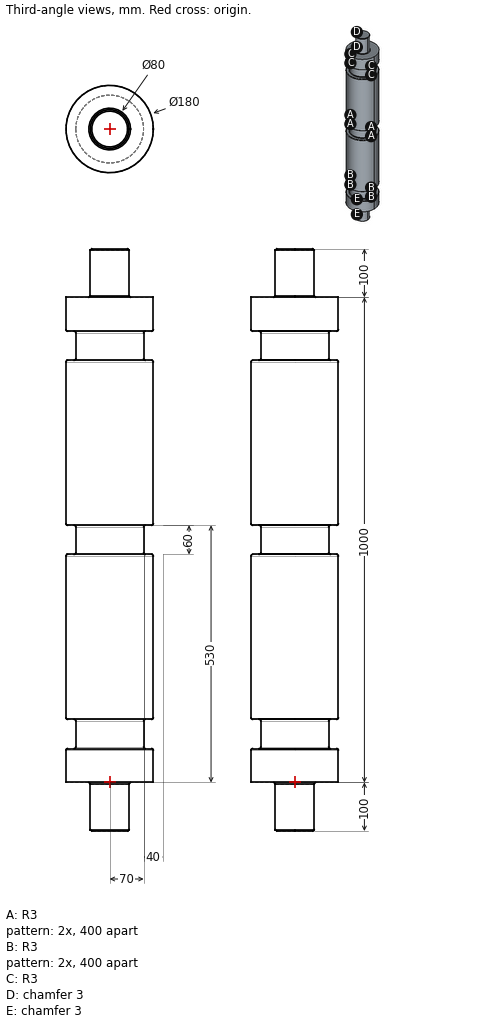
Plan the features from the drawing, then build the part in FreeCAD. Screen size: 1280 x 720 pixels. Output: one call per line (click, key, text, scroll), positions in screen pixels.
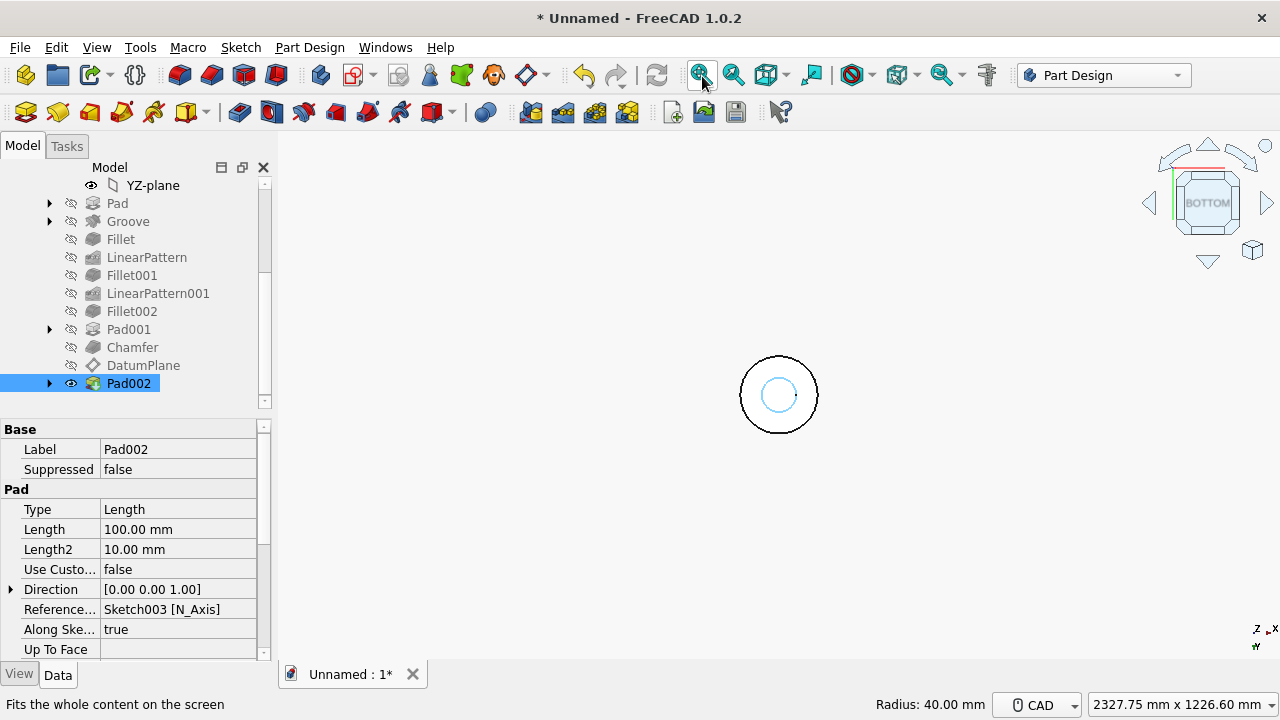
click(702, 76)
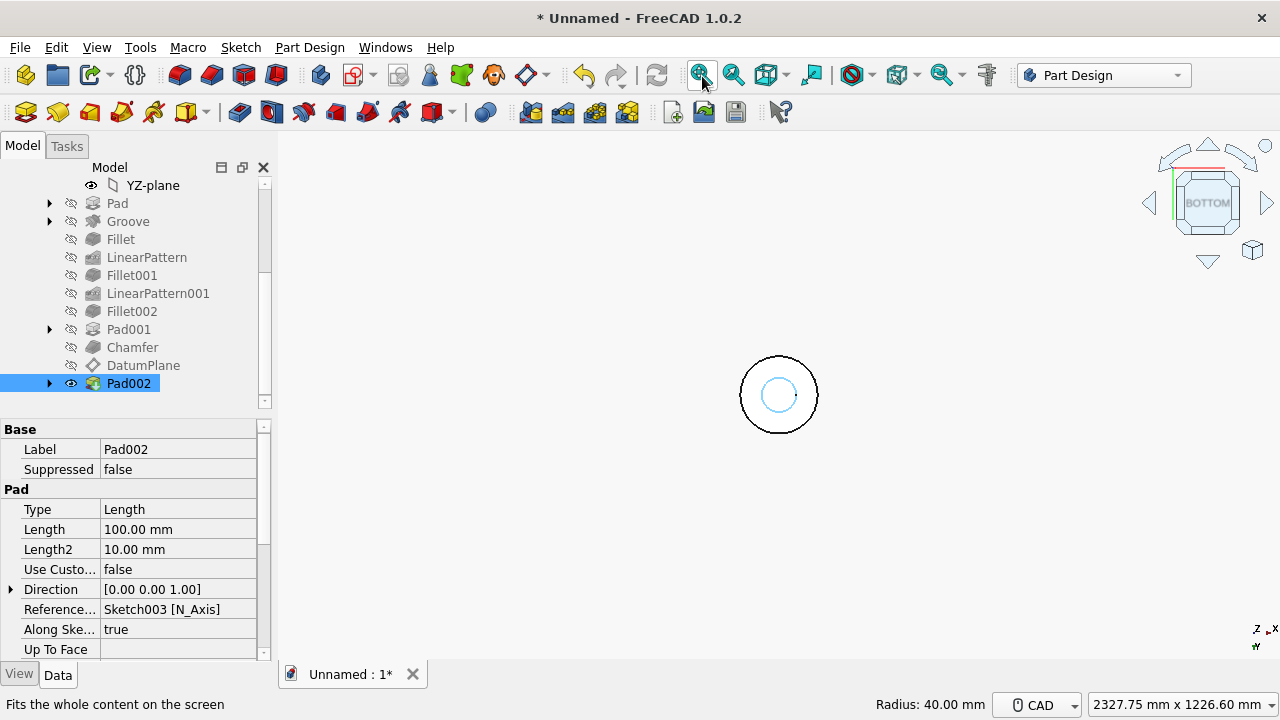
key(4)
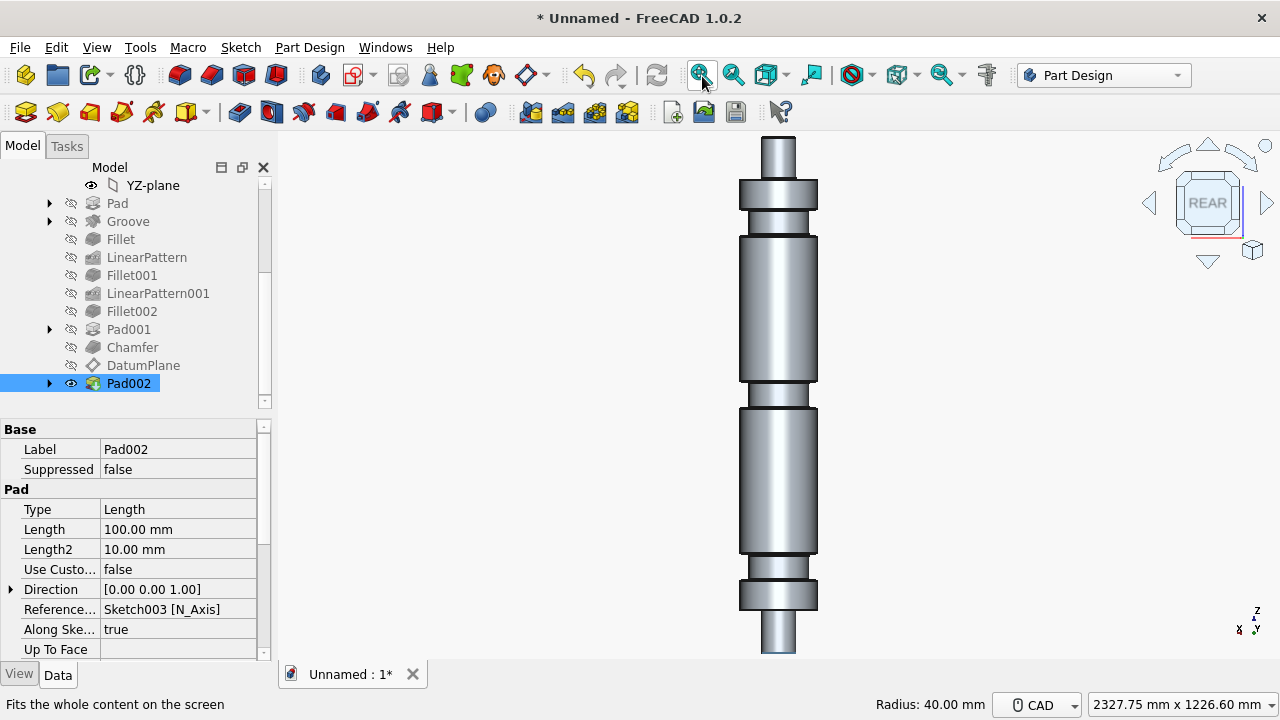
key(6)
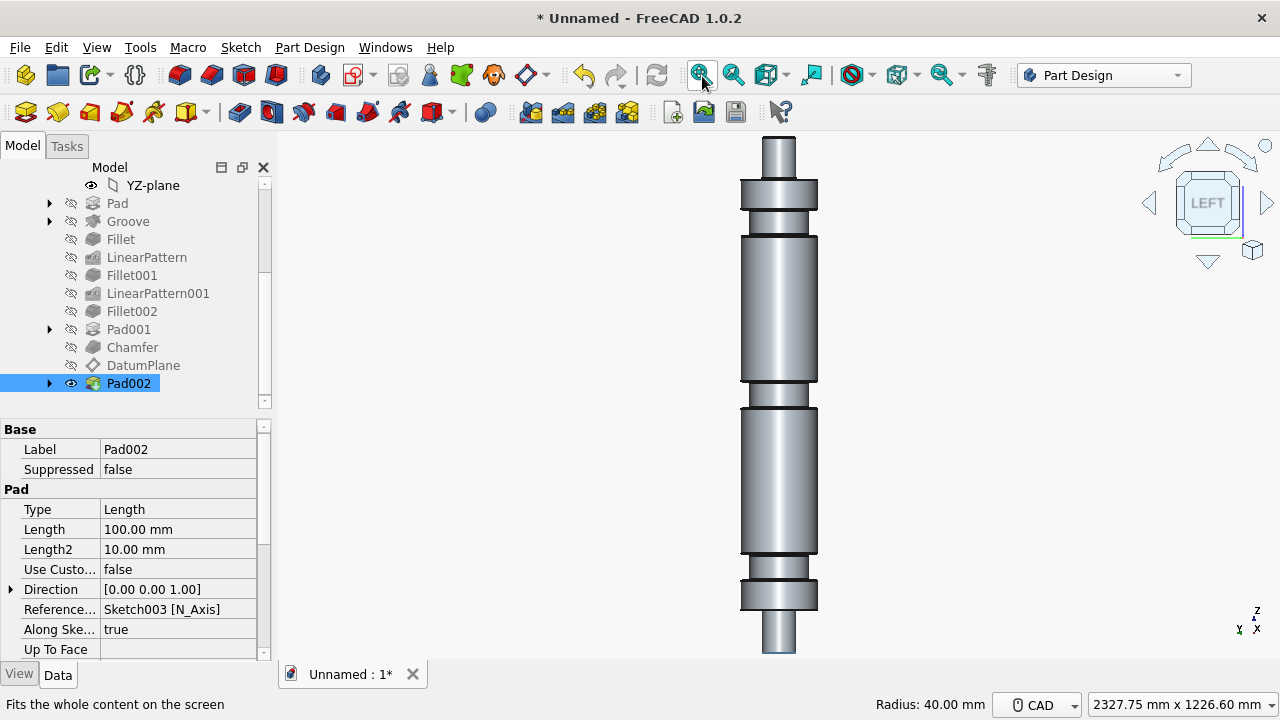
key(v)
key(3)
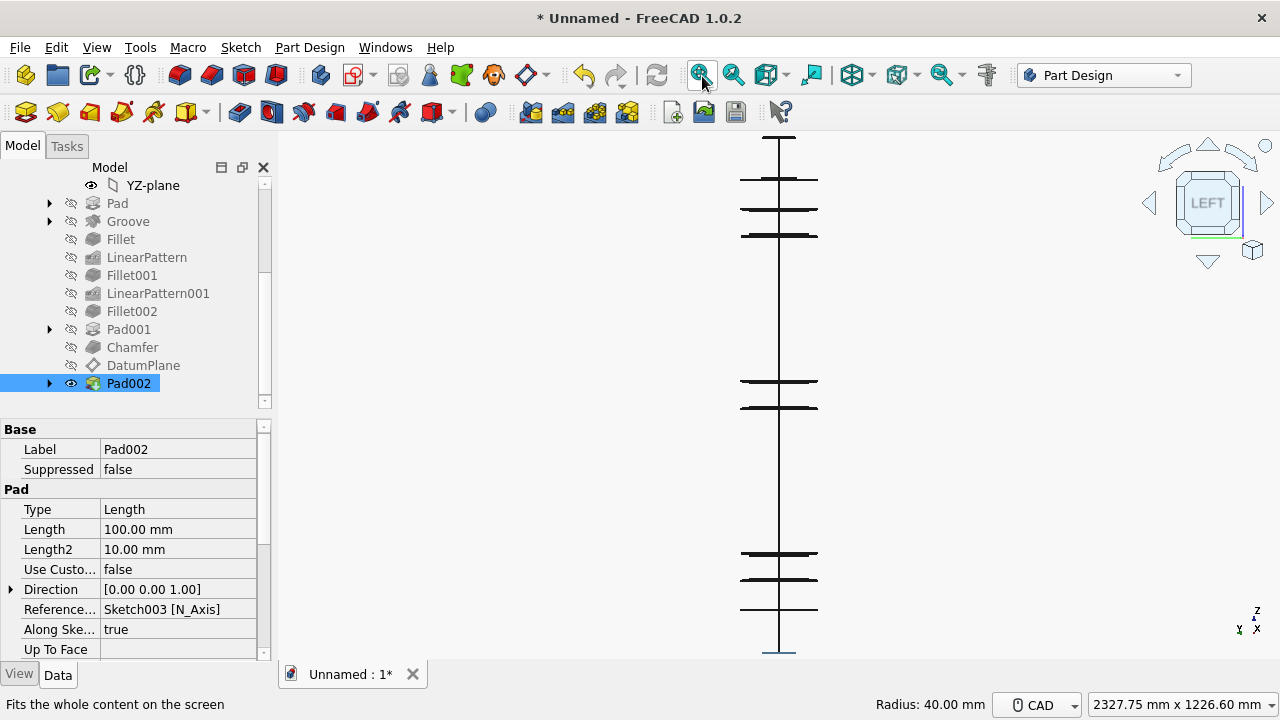
key(0)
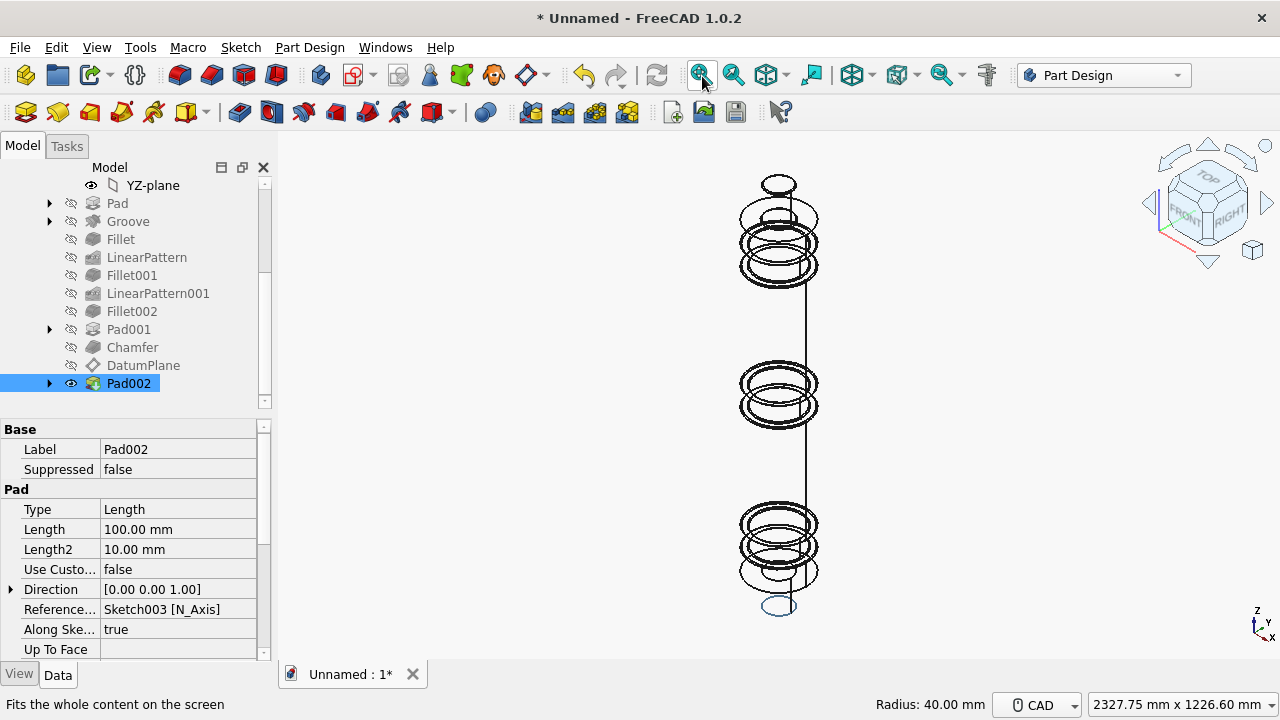
click(764, 574, ctrl)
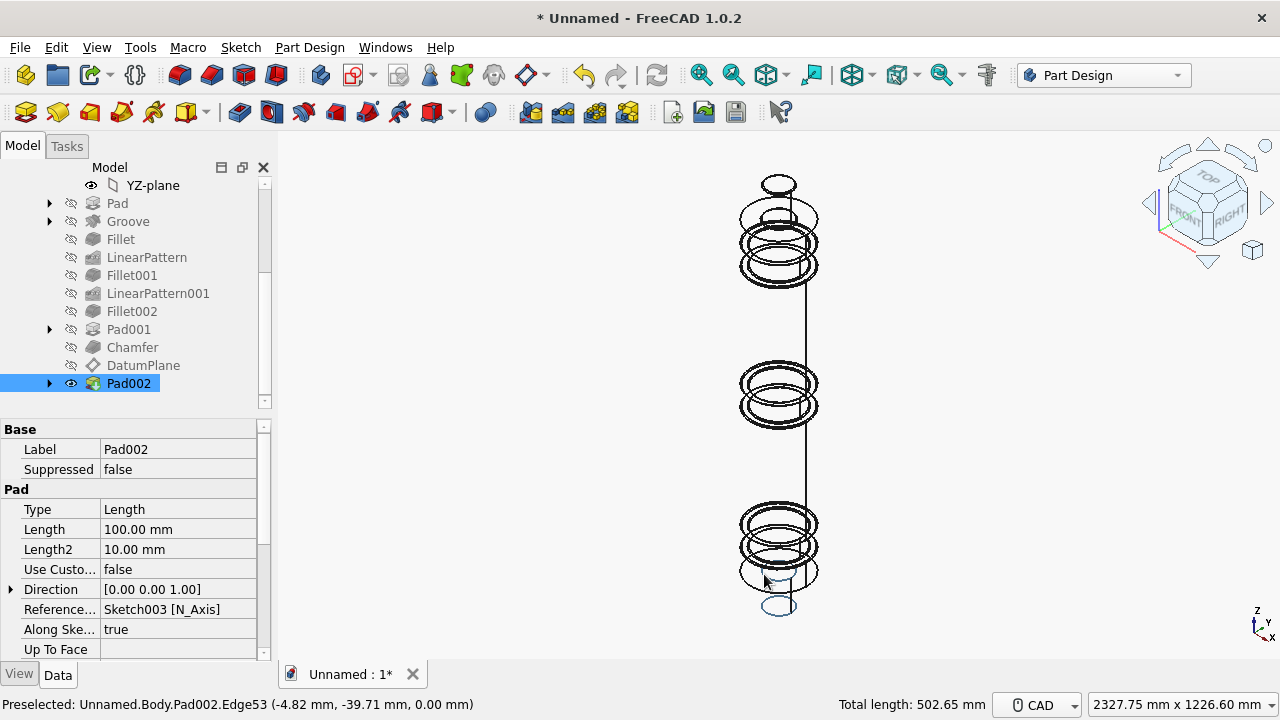
key(v)
key(1)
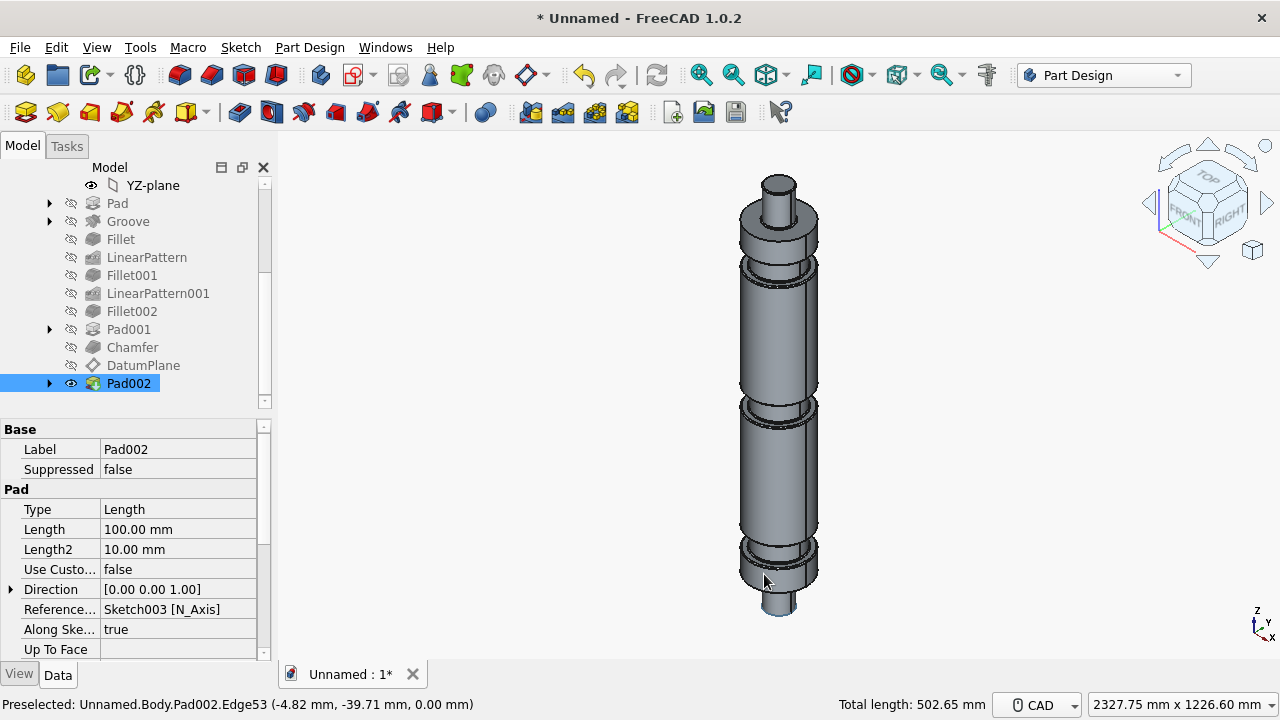
click(212, 76)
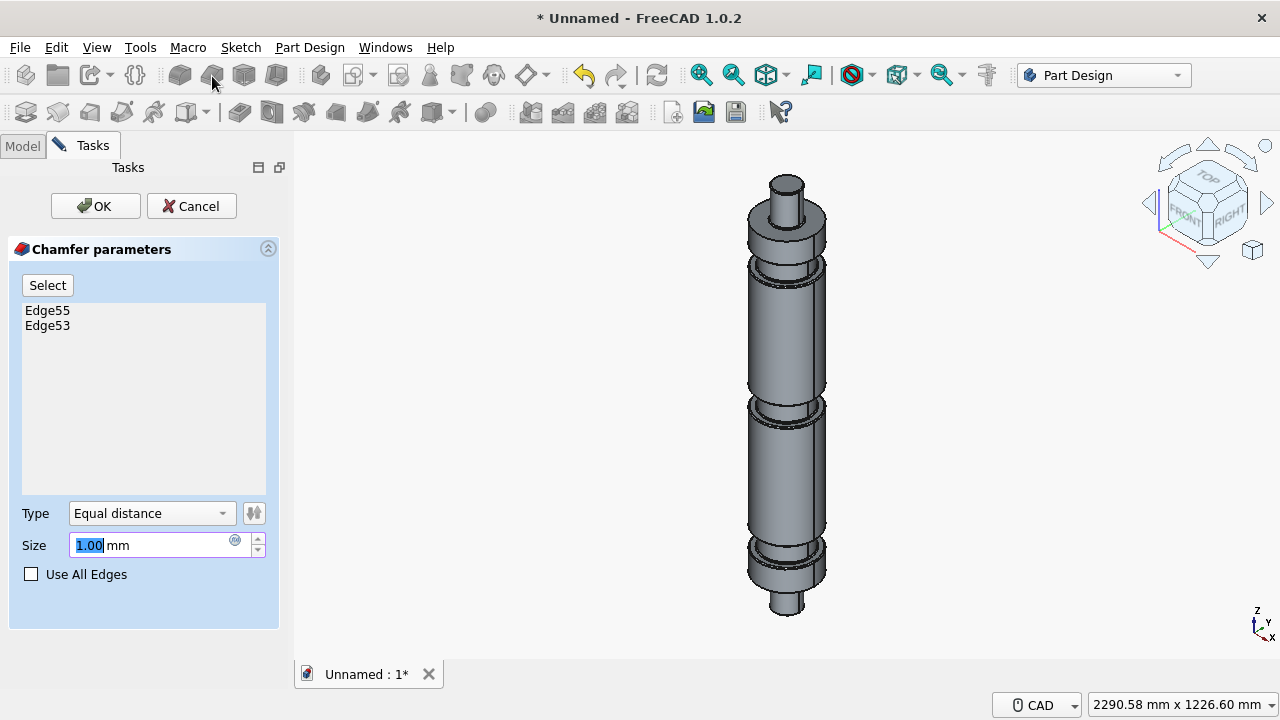
text(3)
key(Tab)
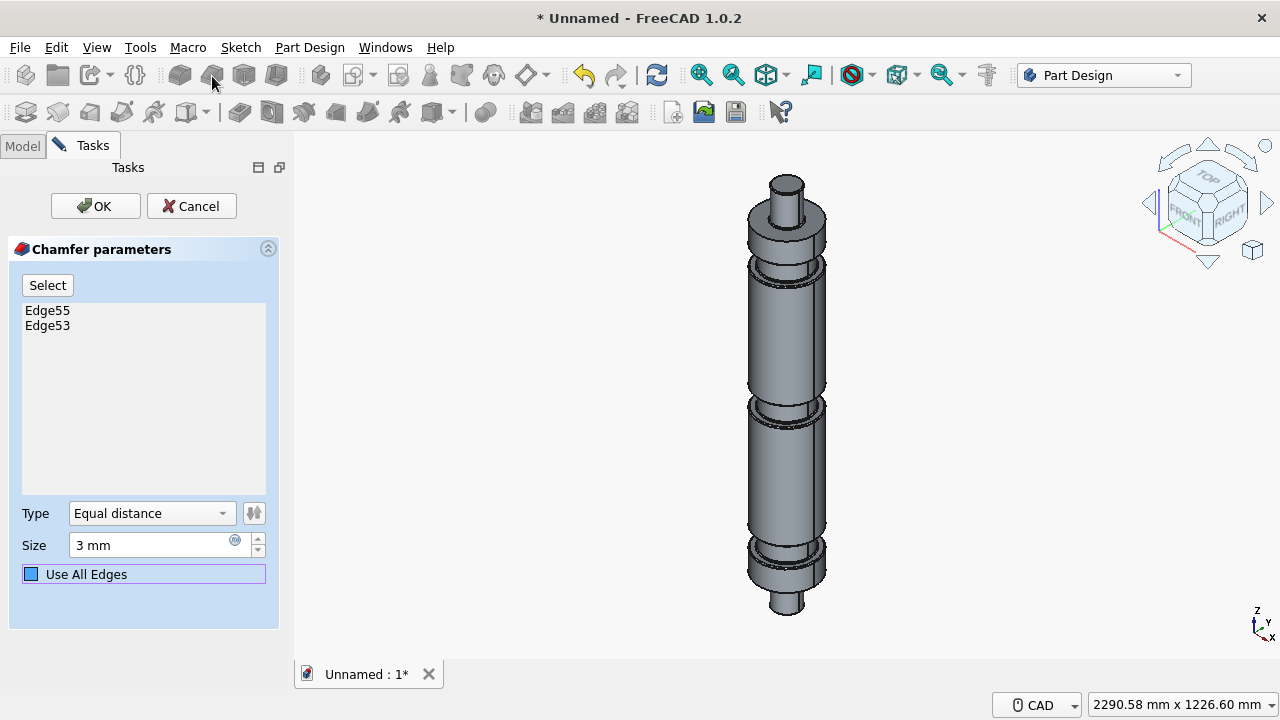
click(96, 206)